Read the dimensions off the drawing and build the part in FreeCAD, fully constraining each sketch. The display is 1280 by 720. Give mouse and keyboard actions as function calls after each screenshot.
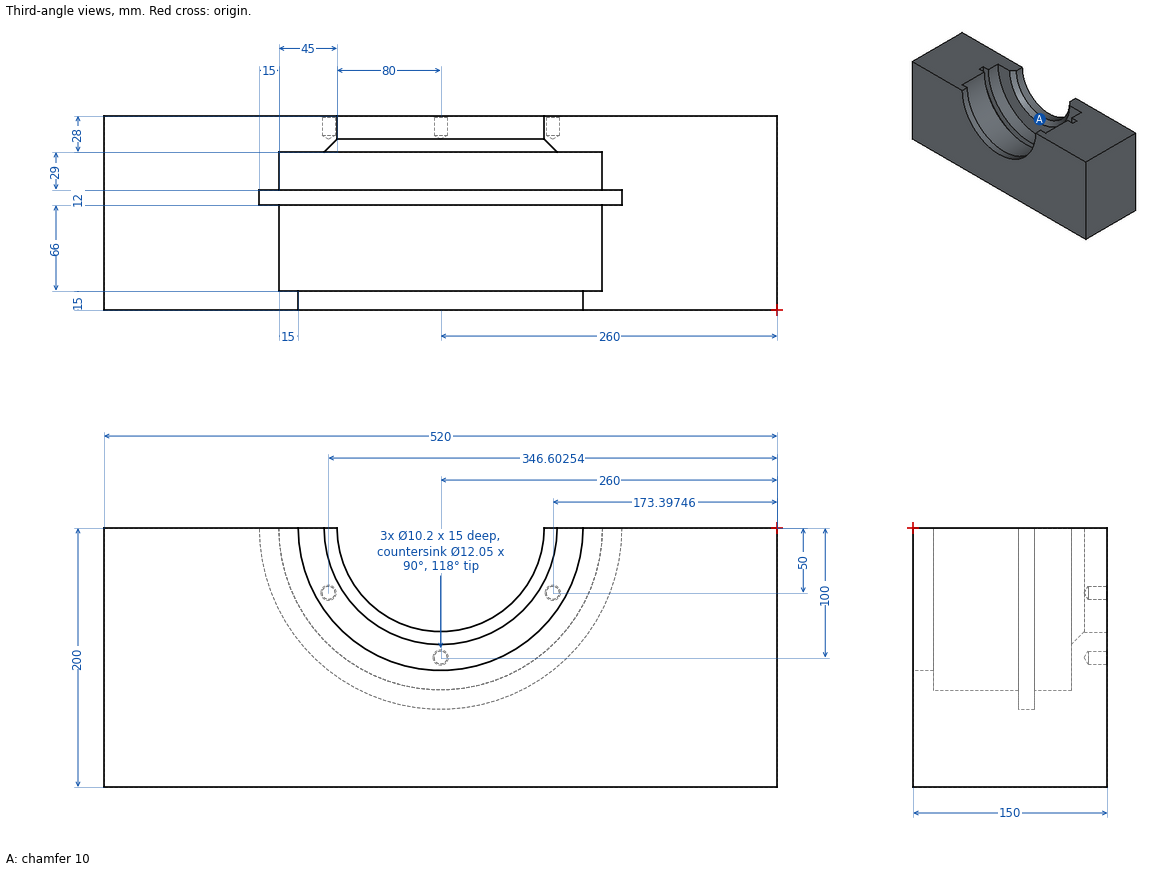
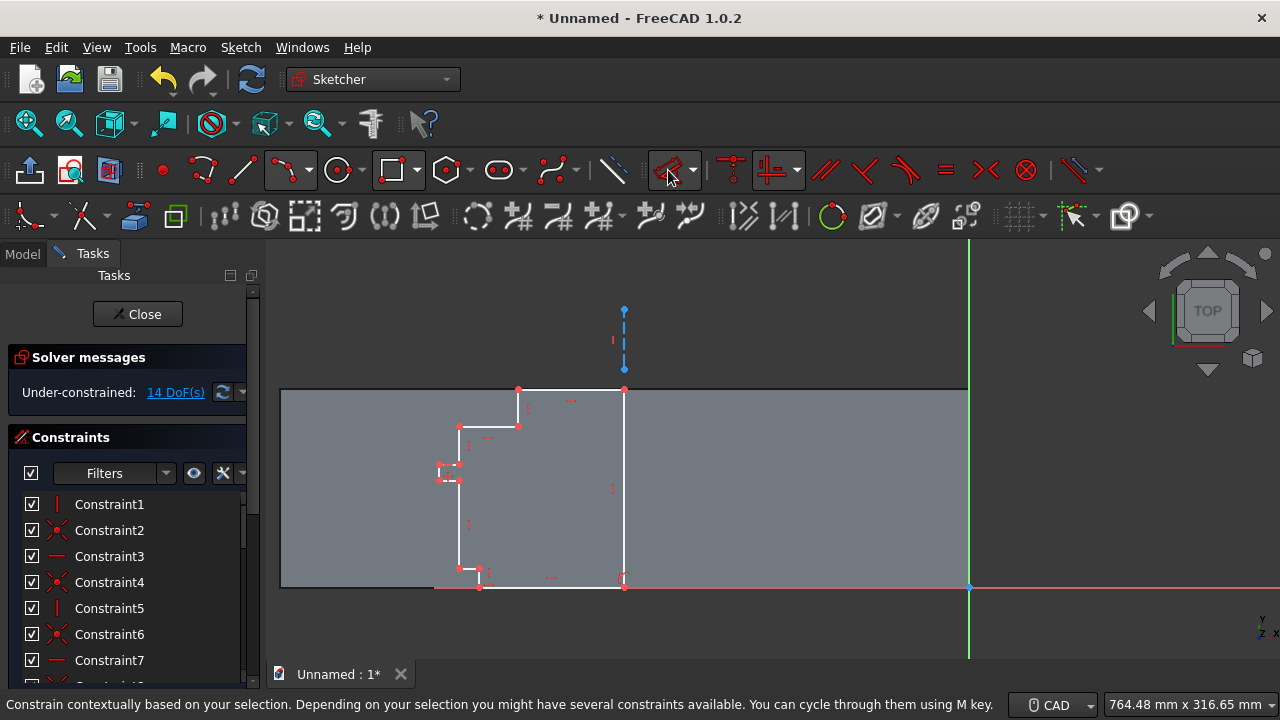
click(592, 390)
click(571, 356)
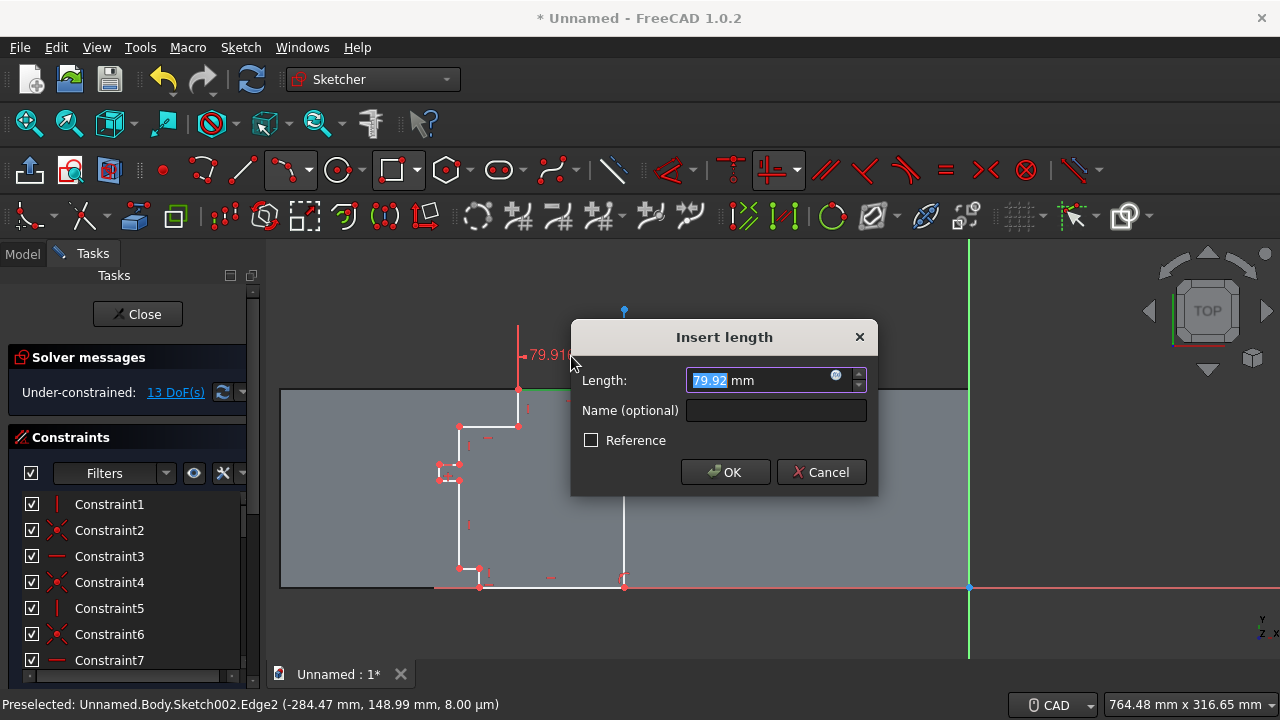
text(80)
key(Return)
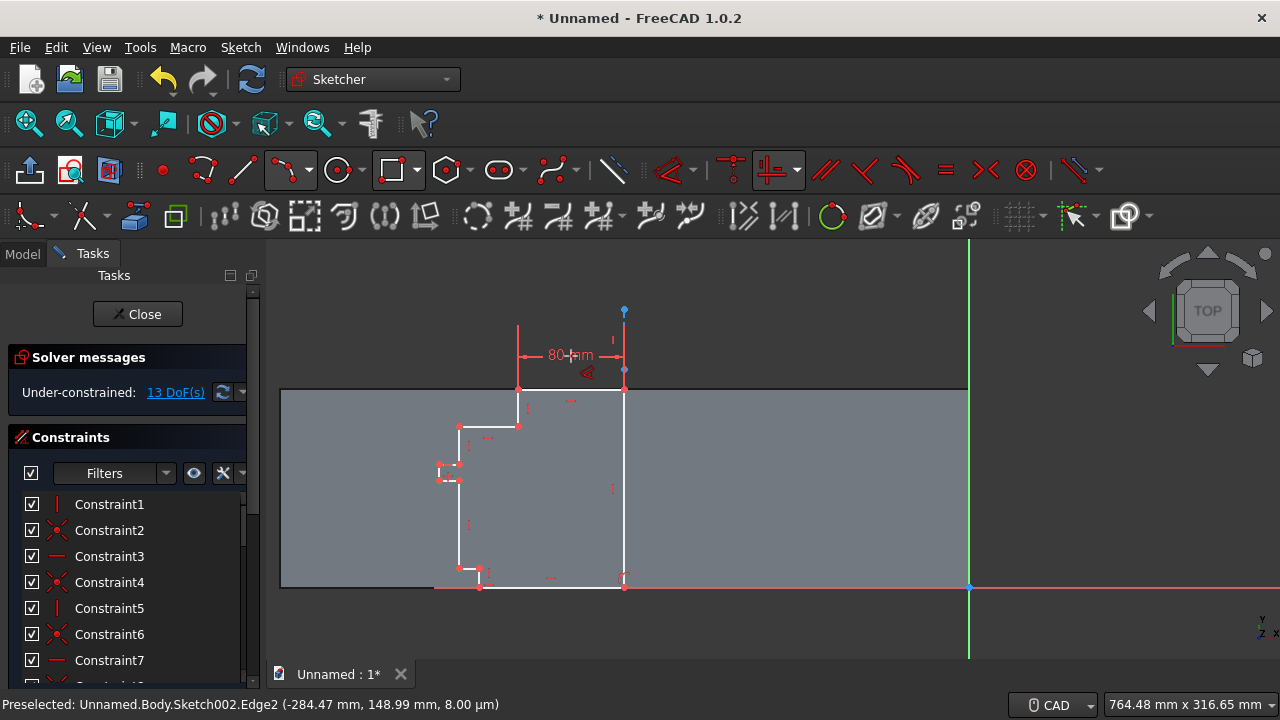
scroll(518, 401, up, 2)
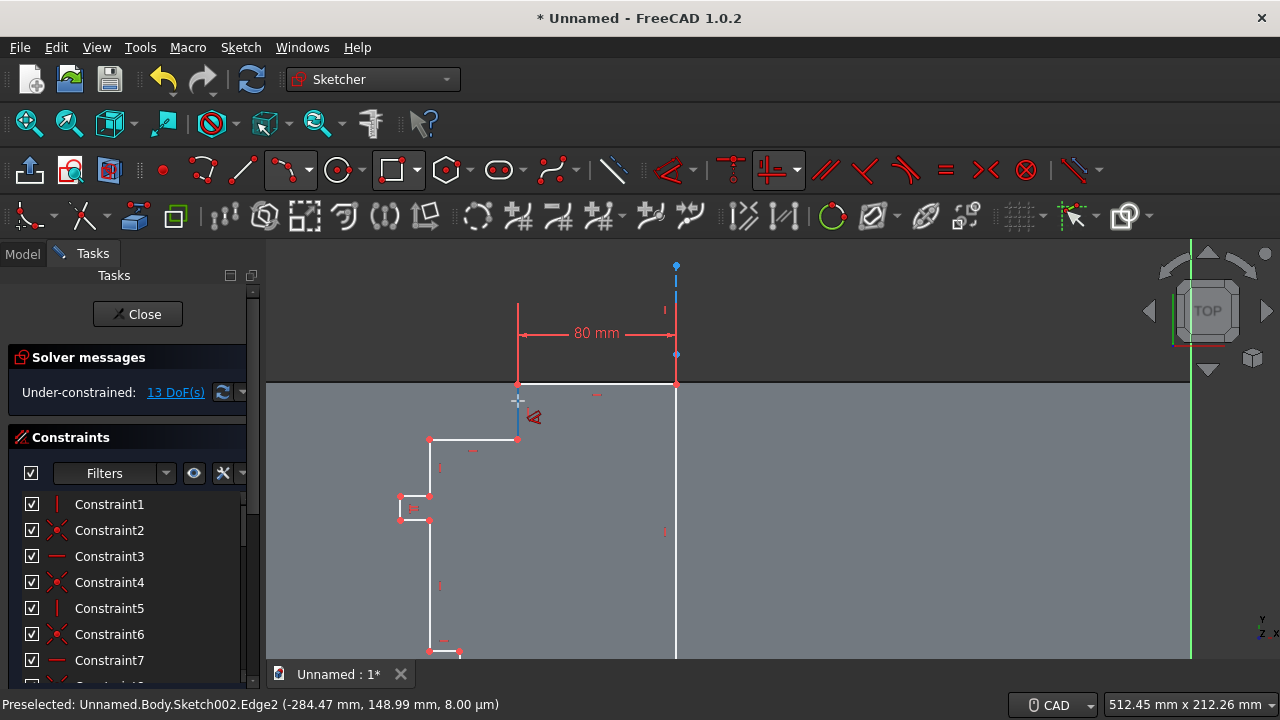
click(518, 401)
click(484, 412)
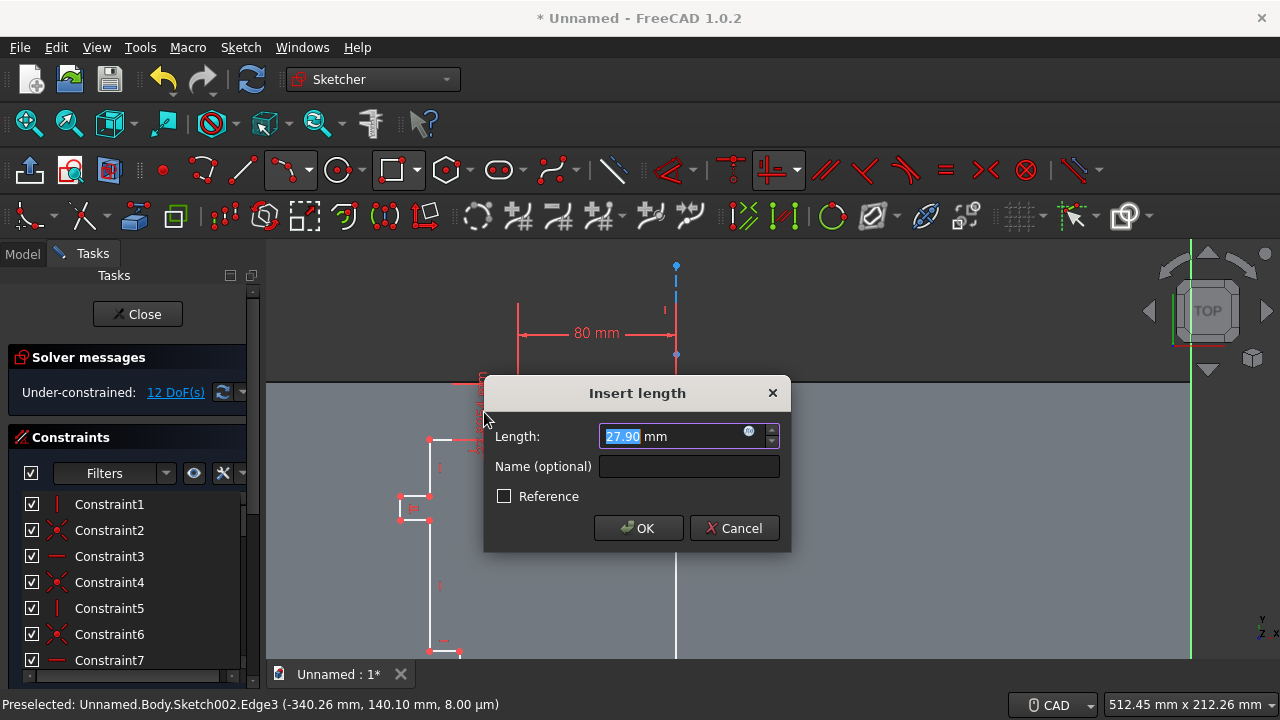
text(28)
key(Return)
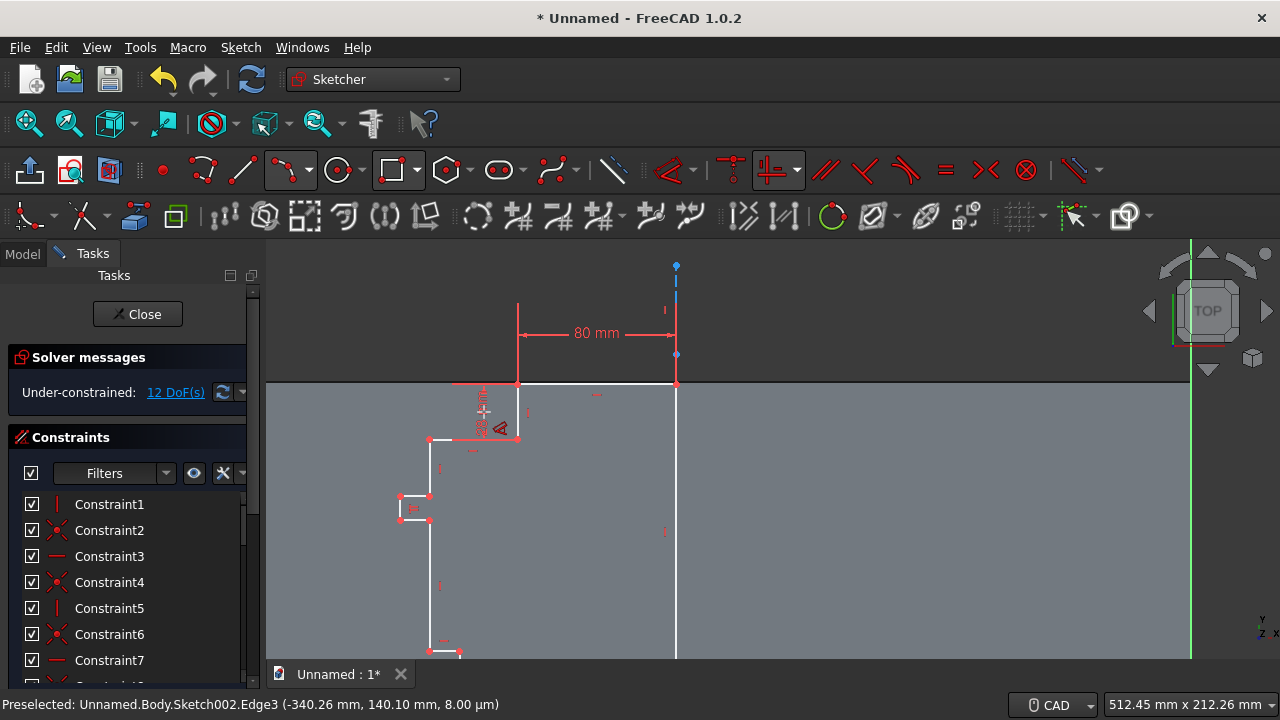
click(491, 440)
click(474, 474)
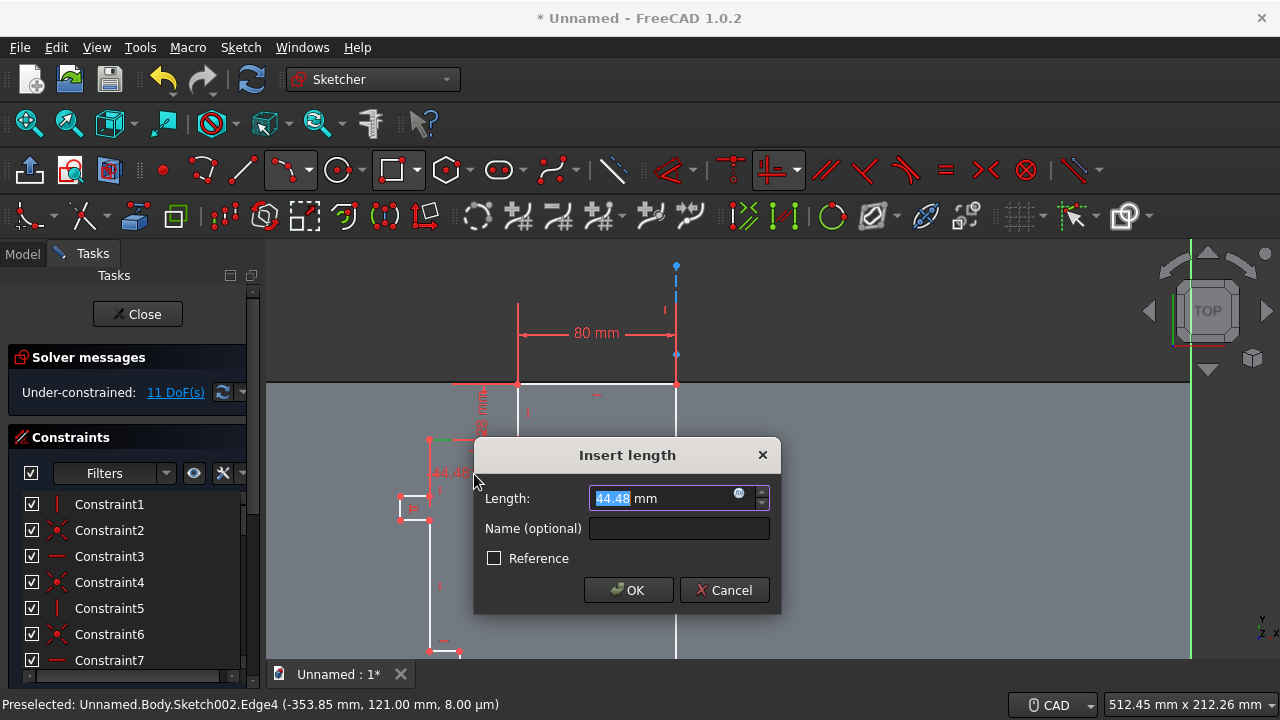
text(45)
key(Return)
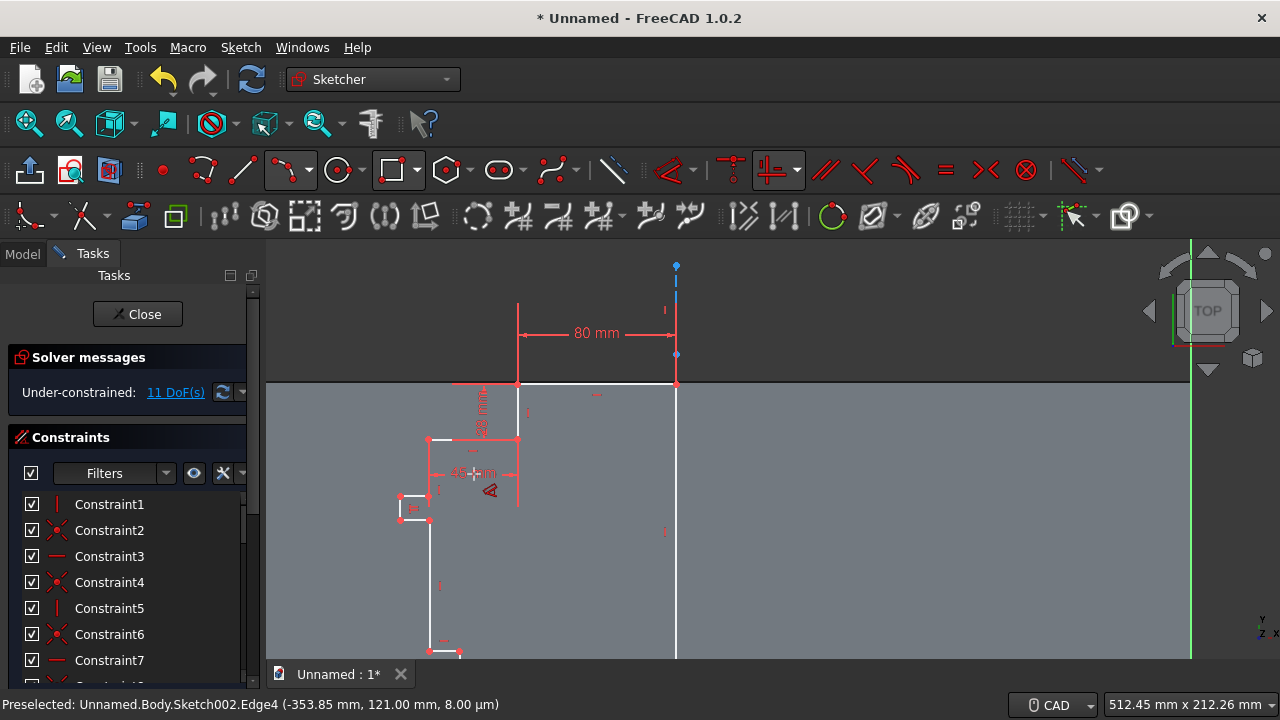
click(429, 457)
click(395, 468)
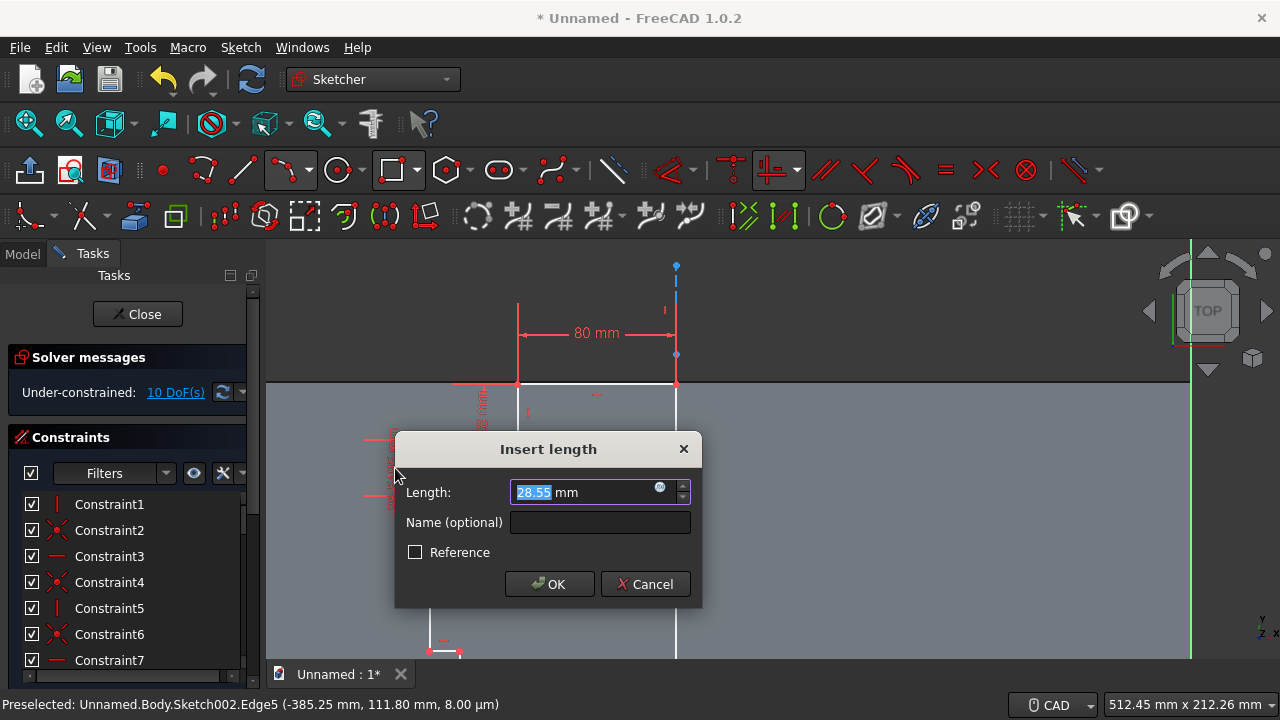
text(29)
key(Return)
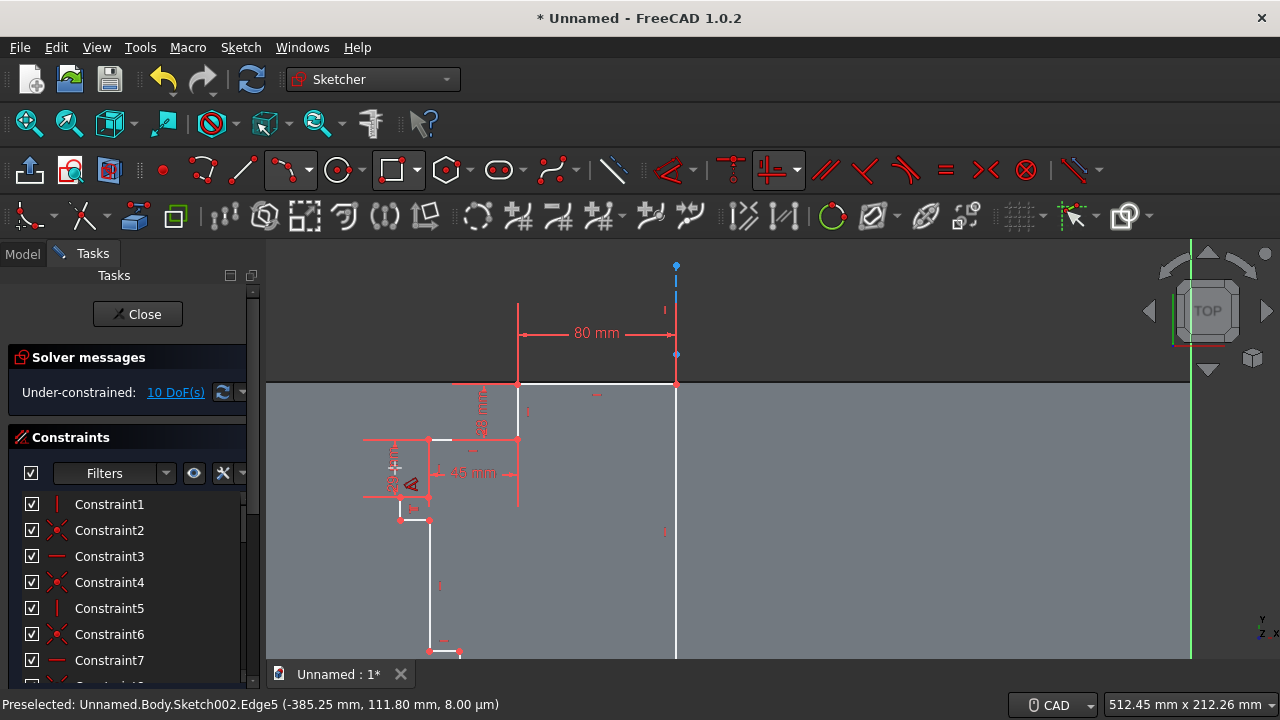
scroll(417, 497, up, 2)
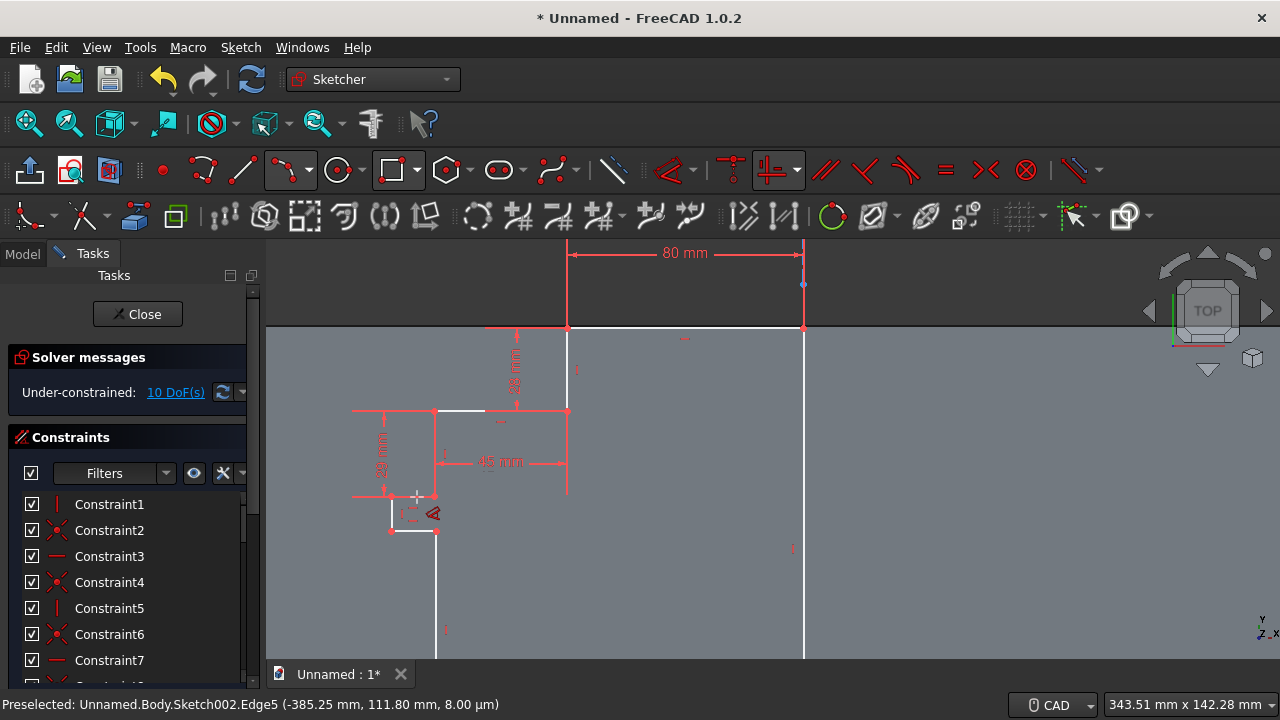
click(417, 497)
click(413, 555)